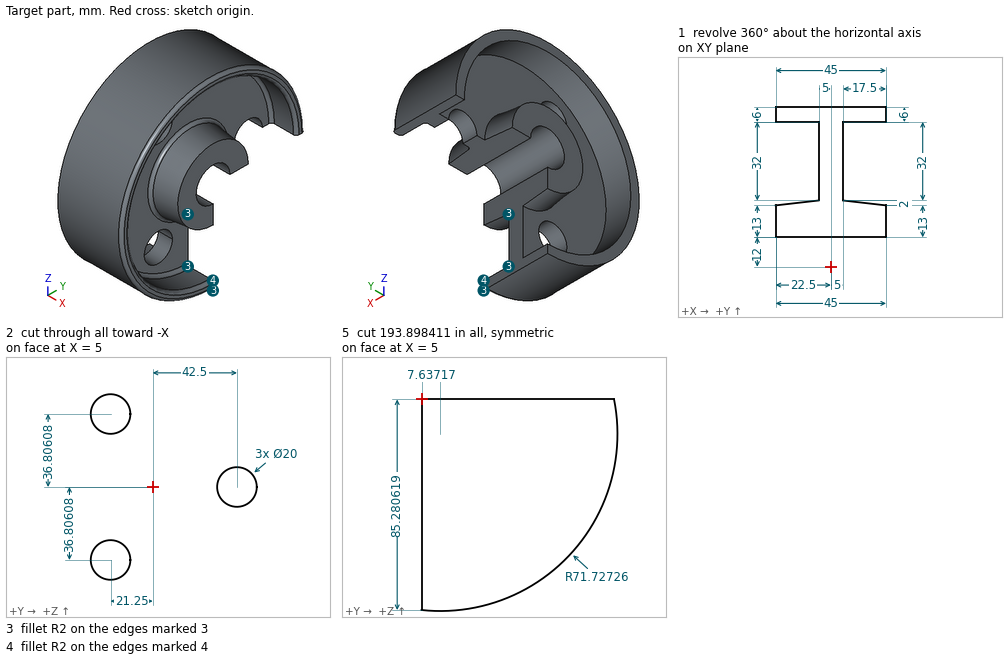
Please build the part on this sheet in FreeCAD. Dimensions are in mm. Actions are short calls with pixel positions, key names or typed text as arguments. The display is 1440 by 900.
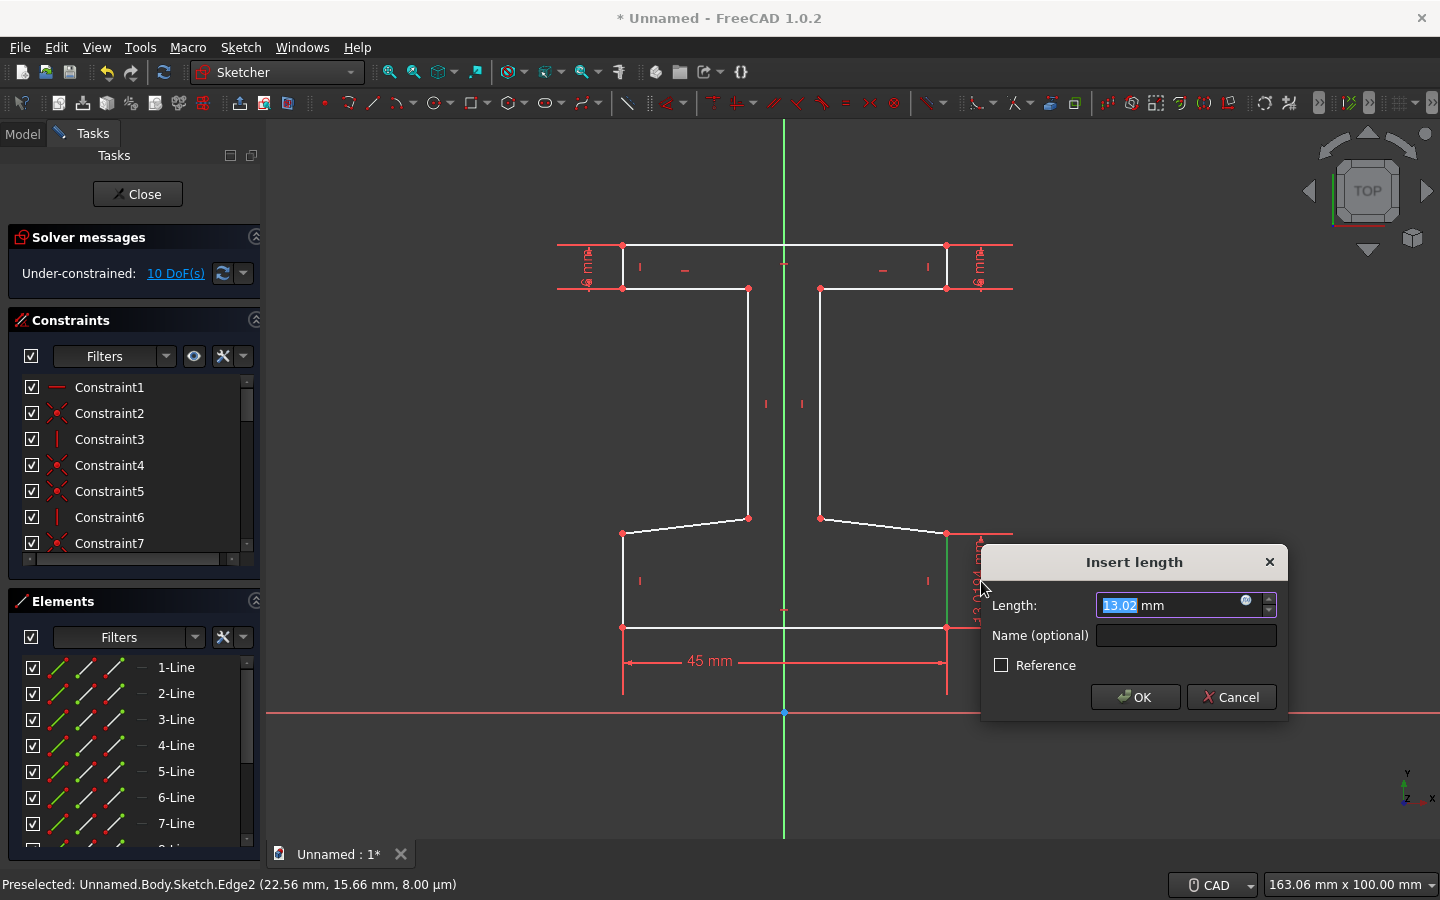
text(13)
key(Return)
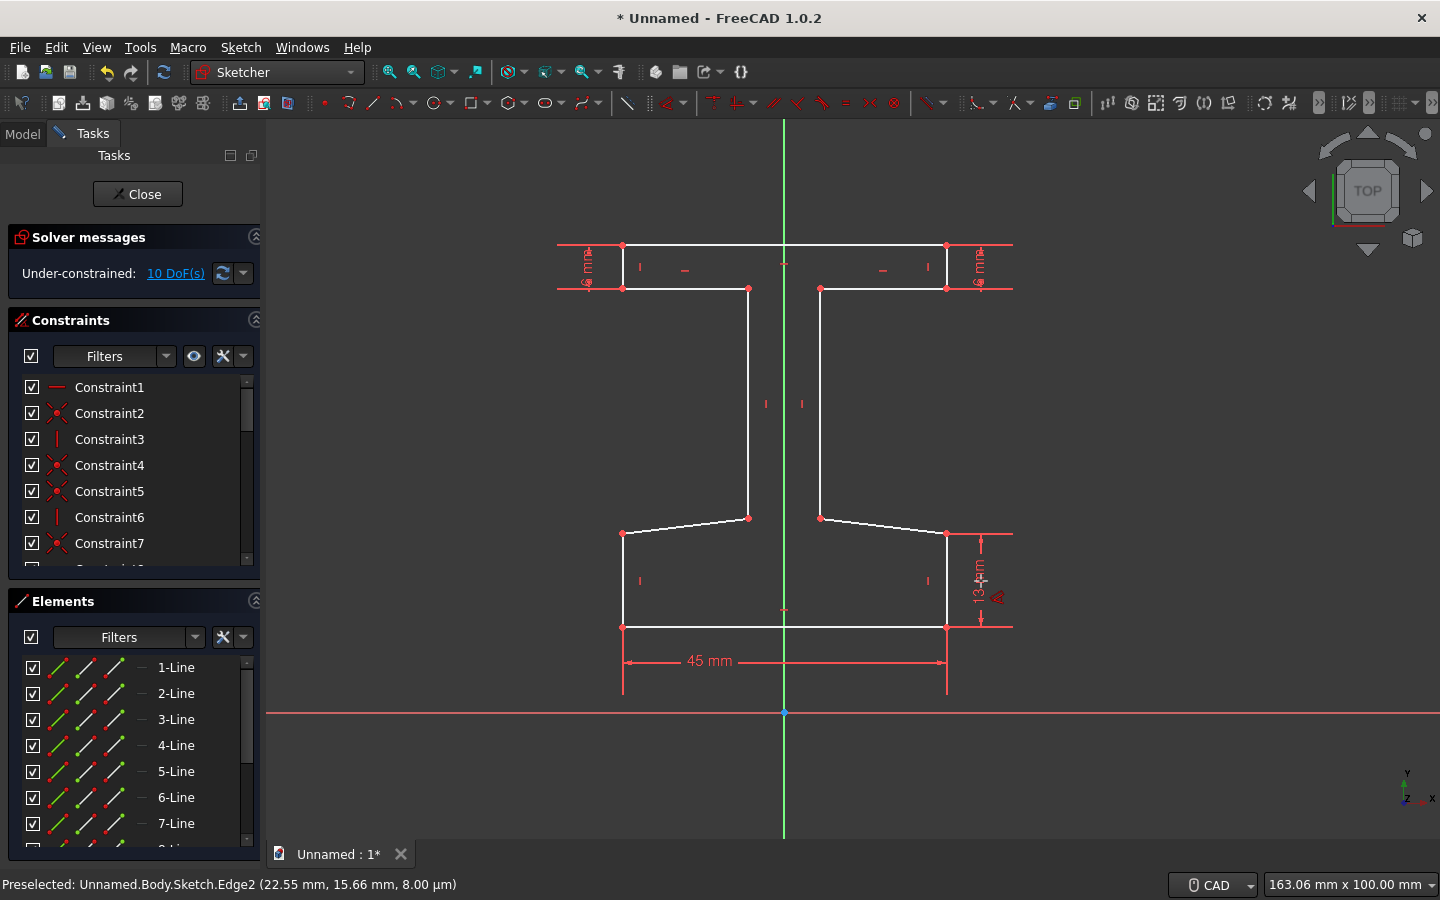
click(820, 450)
click(854, 404)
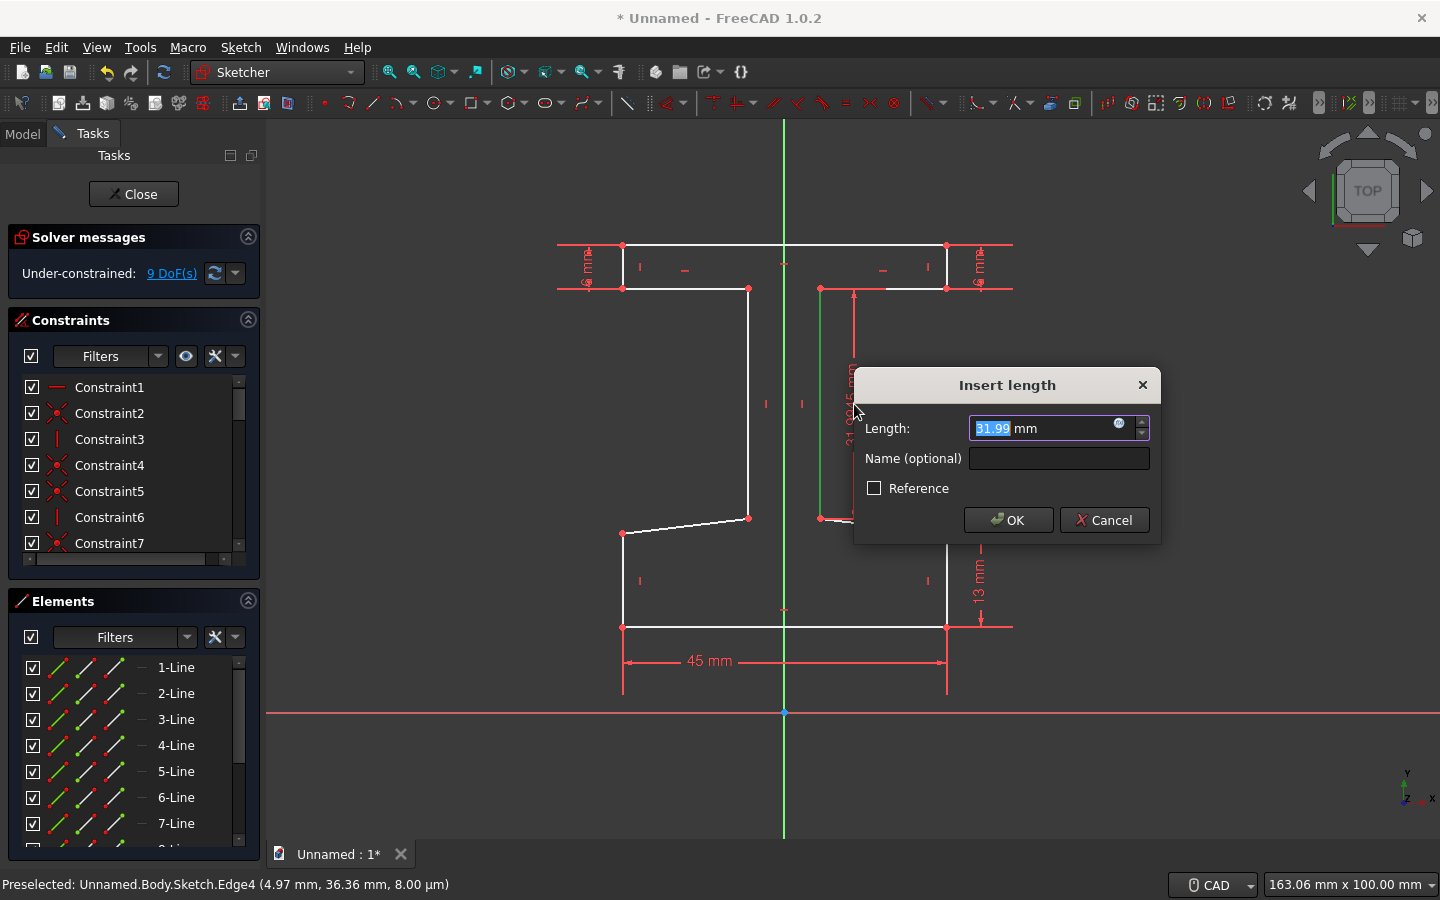
text(32)
key(Return)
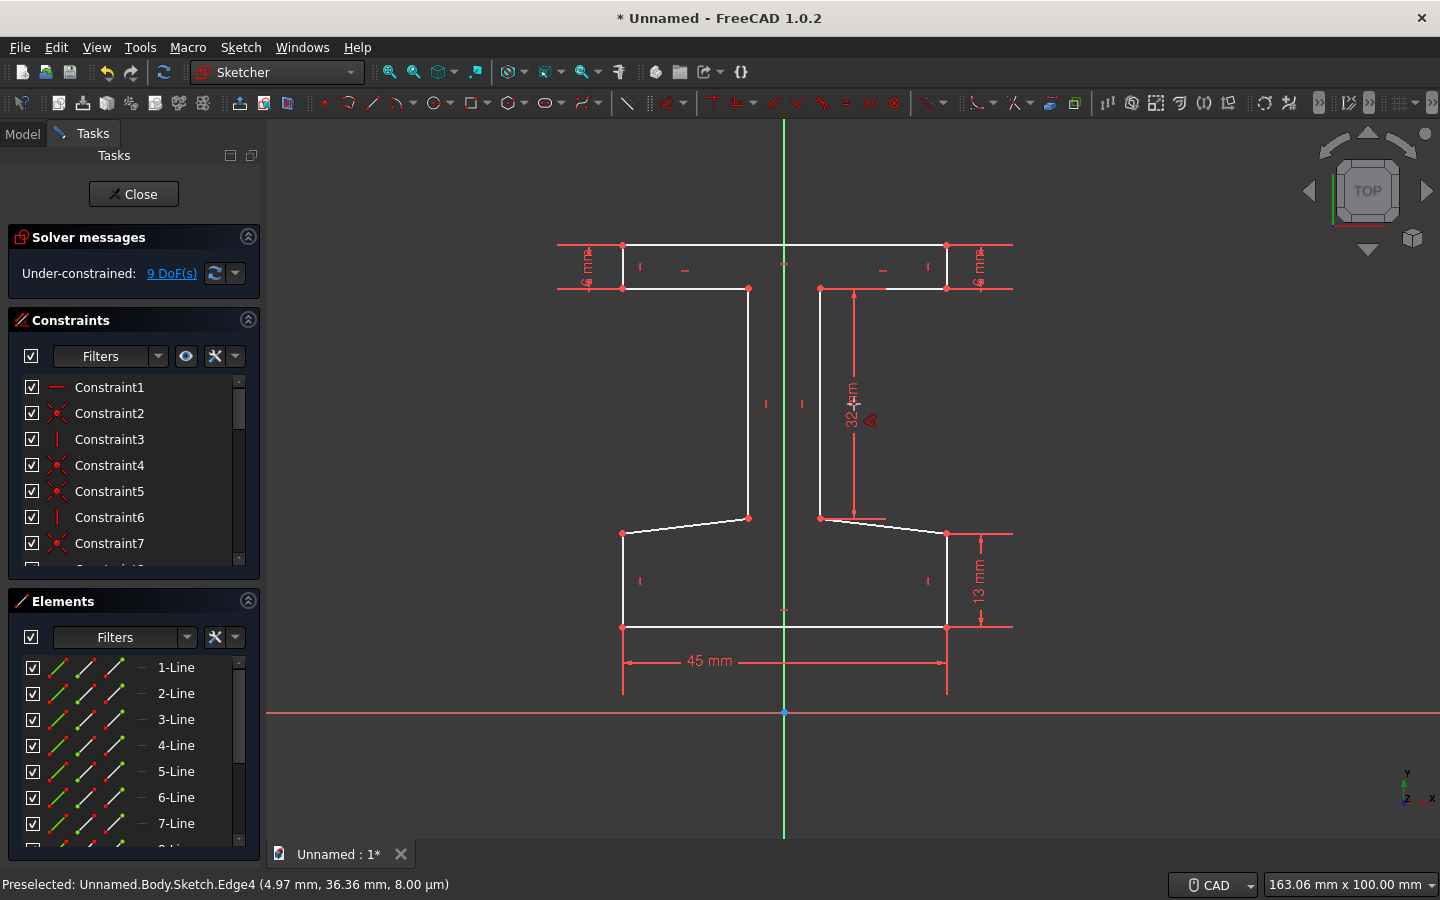
click(850, 245)
click(710, 211)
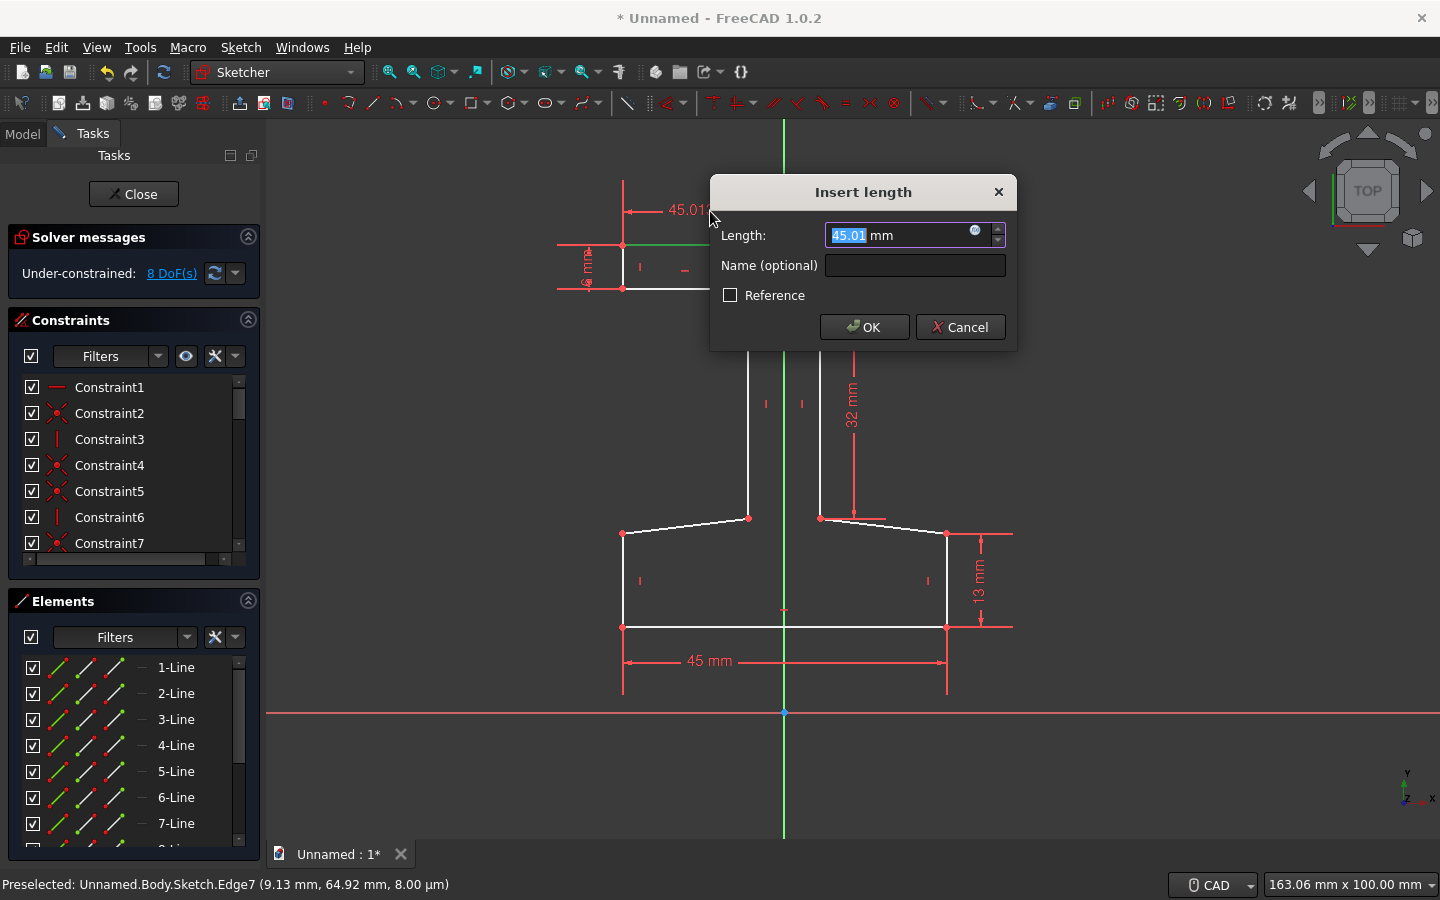
text(45)
key(Return)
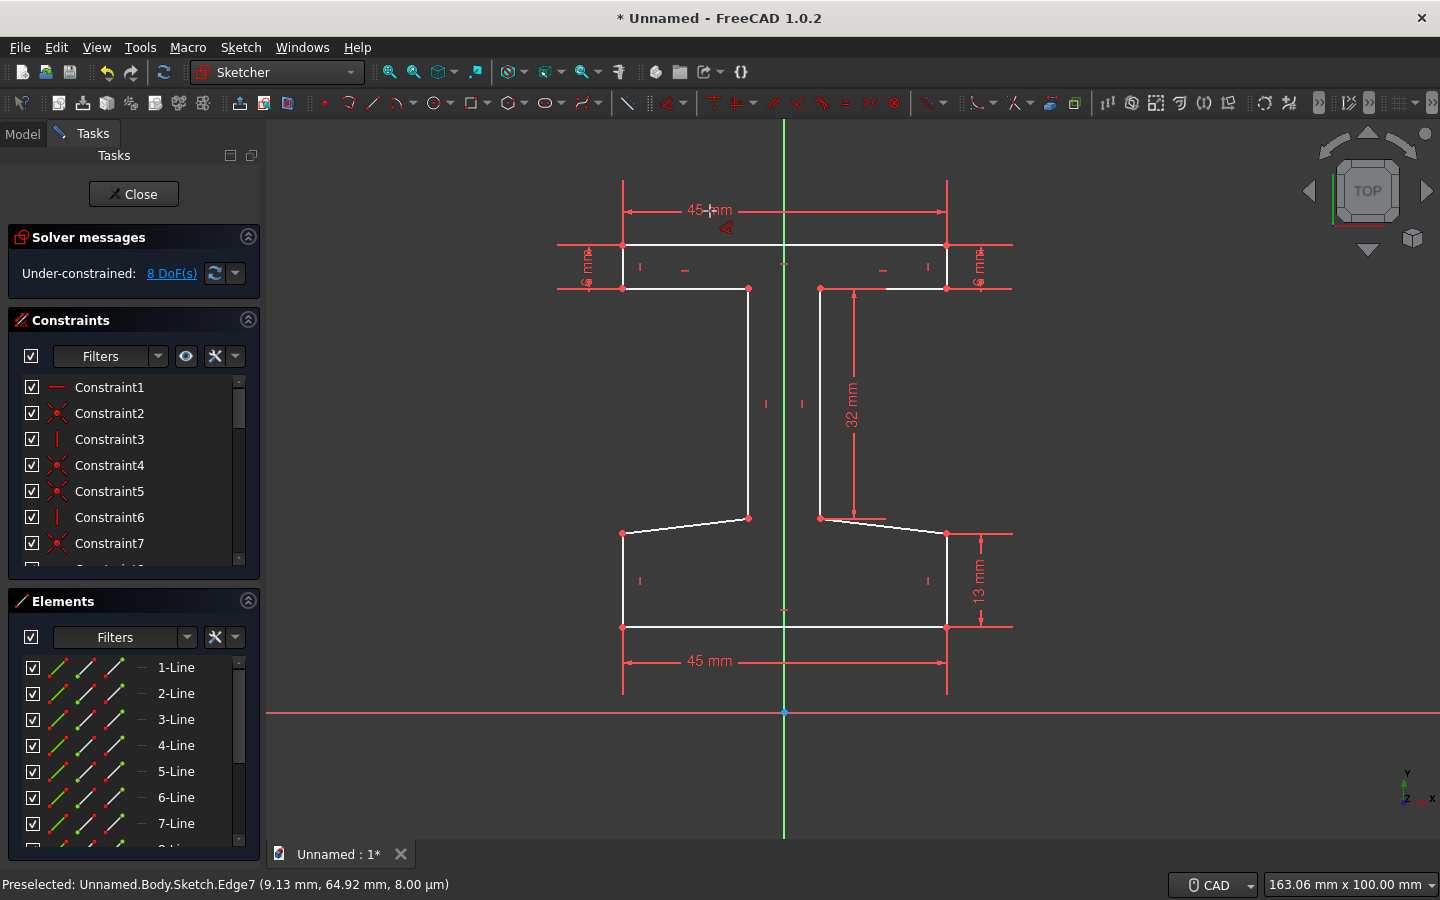
click(748, 358)
click(714, 404)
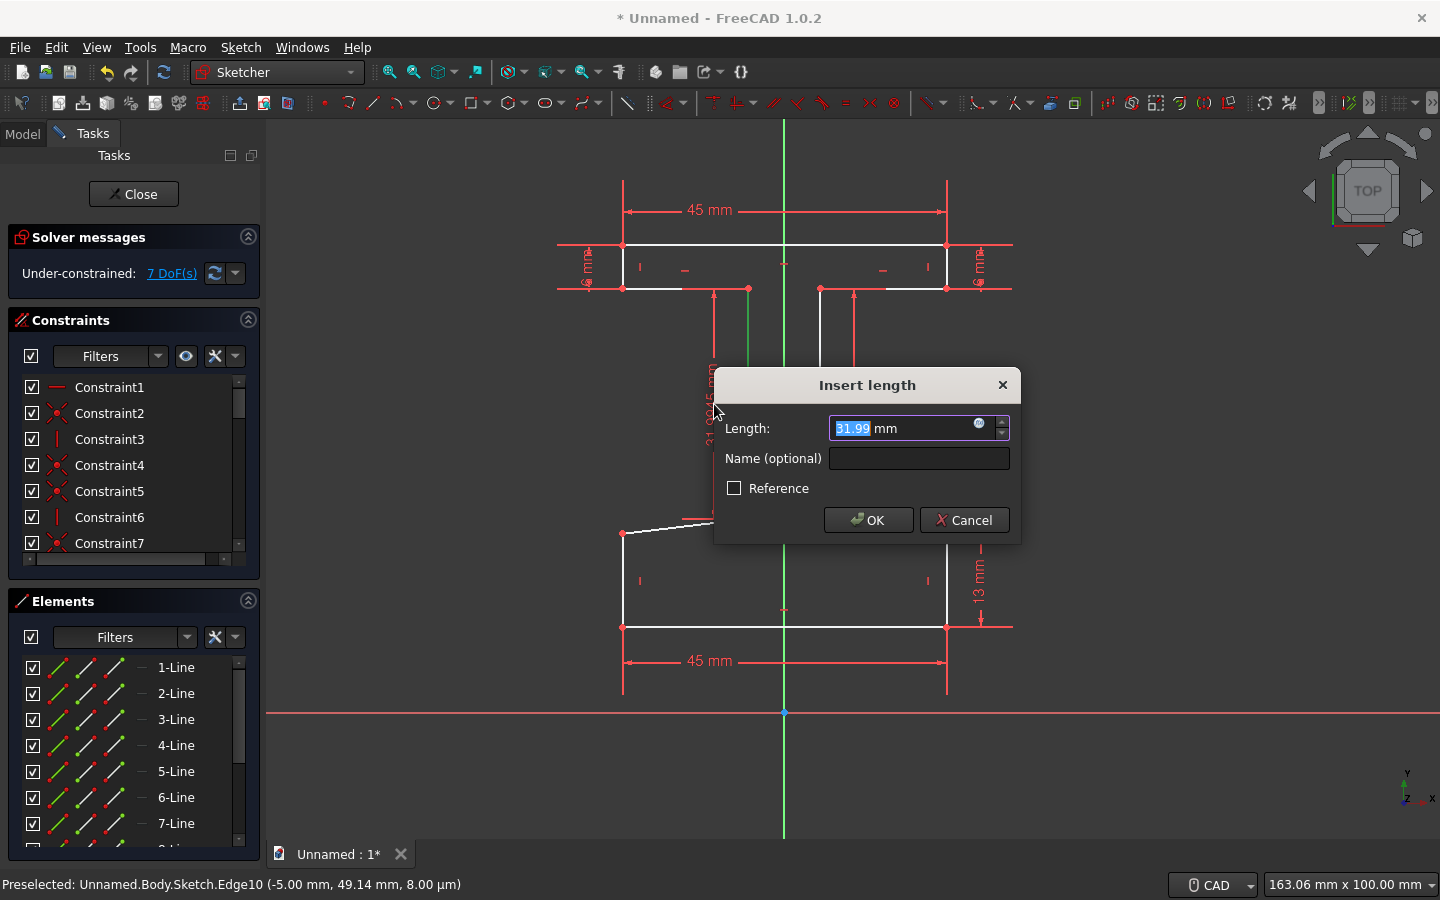
text(32)
key(Return)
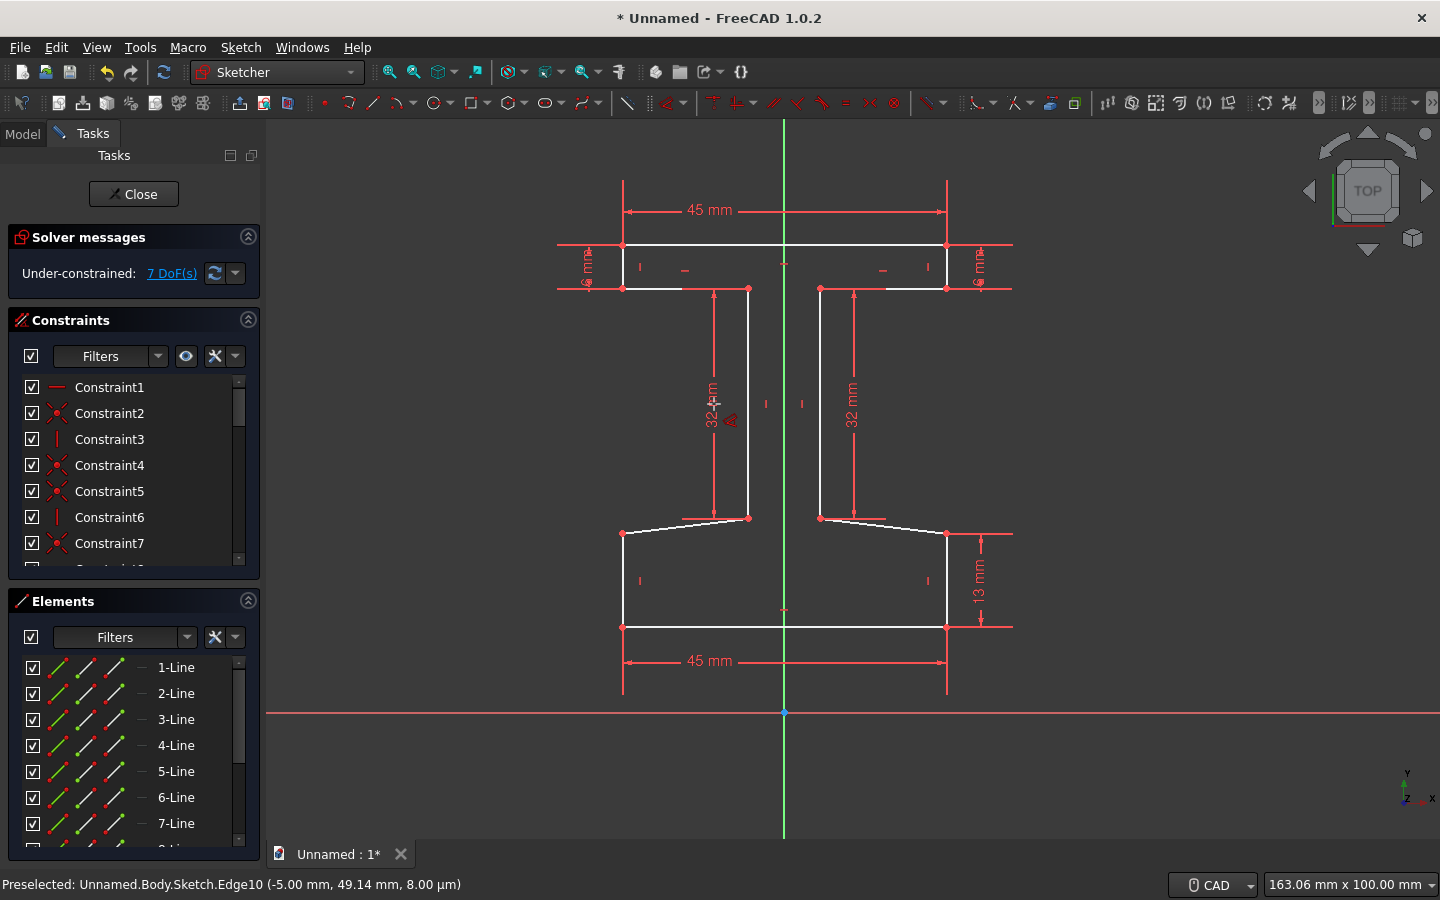
click(623, 562)
click(589, 581)